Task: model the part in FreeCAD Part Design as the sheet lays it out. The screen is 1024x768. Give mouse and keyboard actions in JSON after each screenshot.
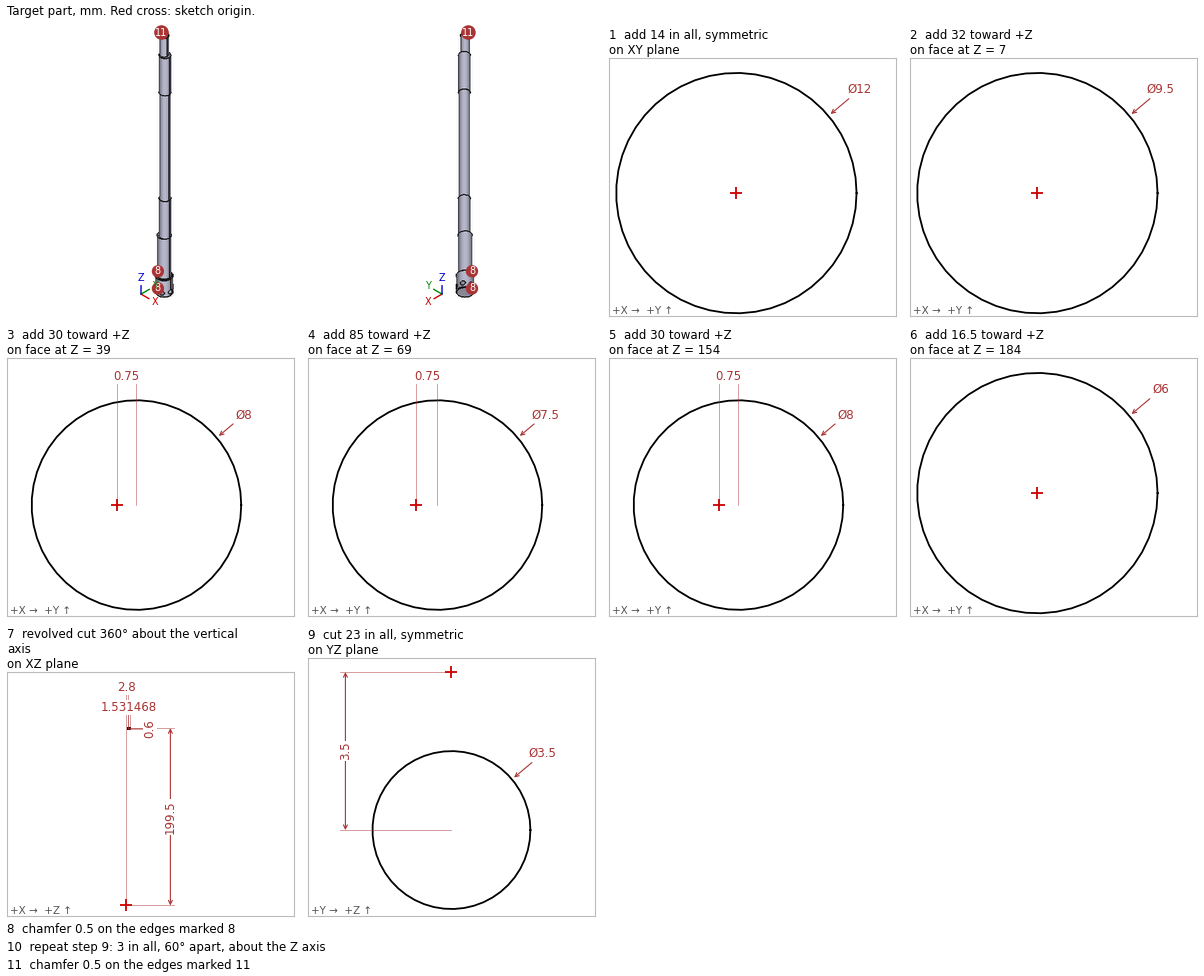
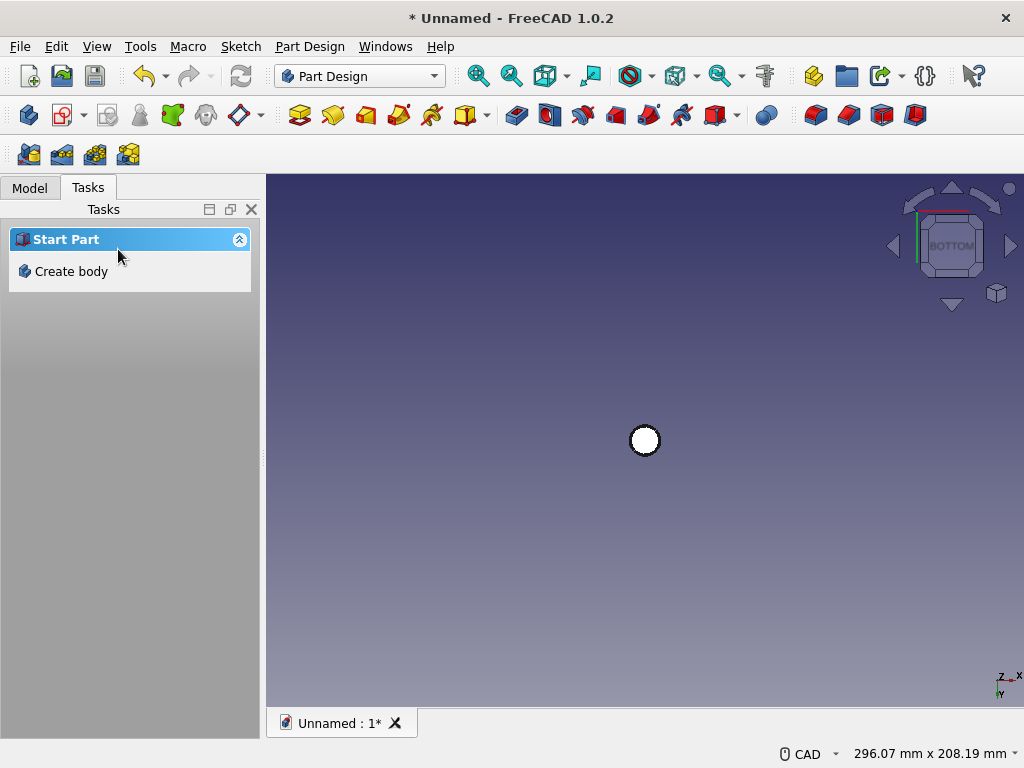
{"action": "key", "text": "v f"}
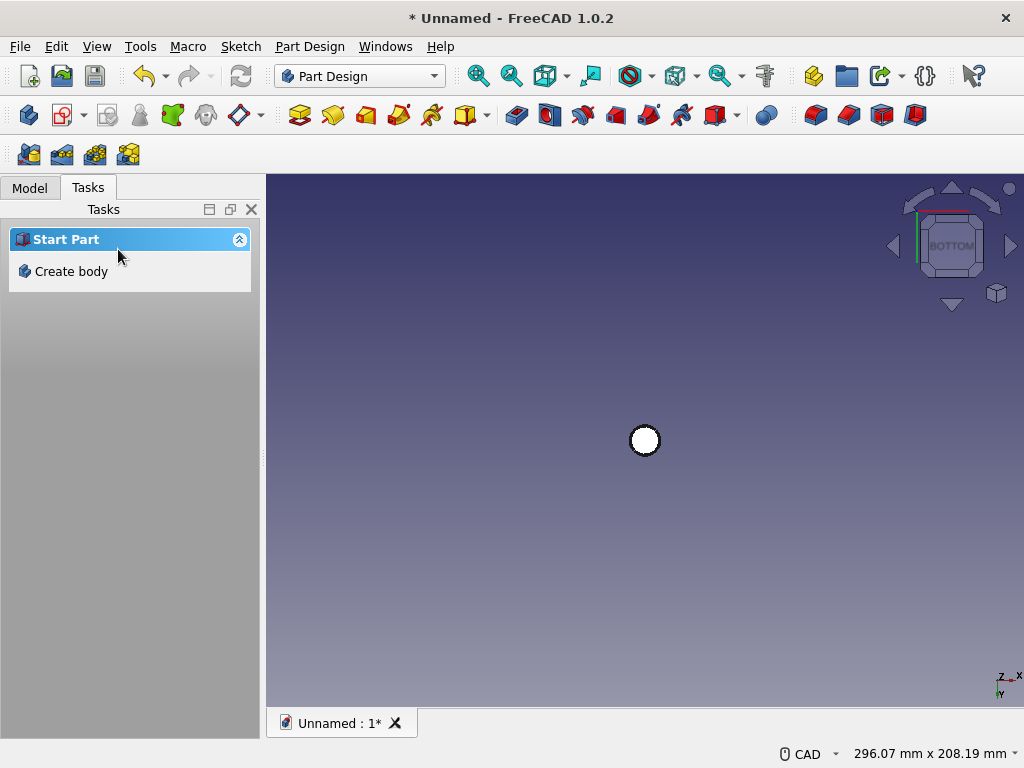
{"action": "left_click", "coordinate": [30, 188]}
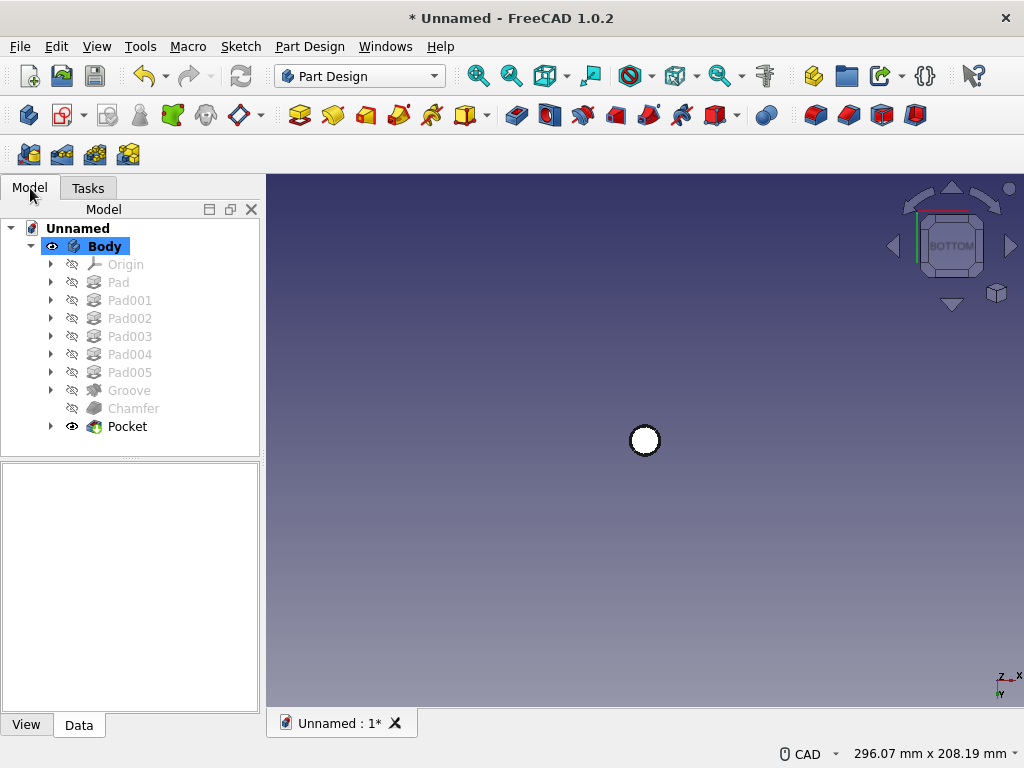
{"action": "left_click", "coordinate": [117, 426]}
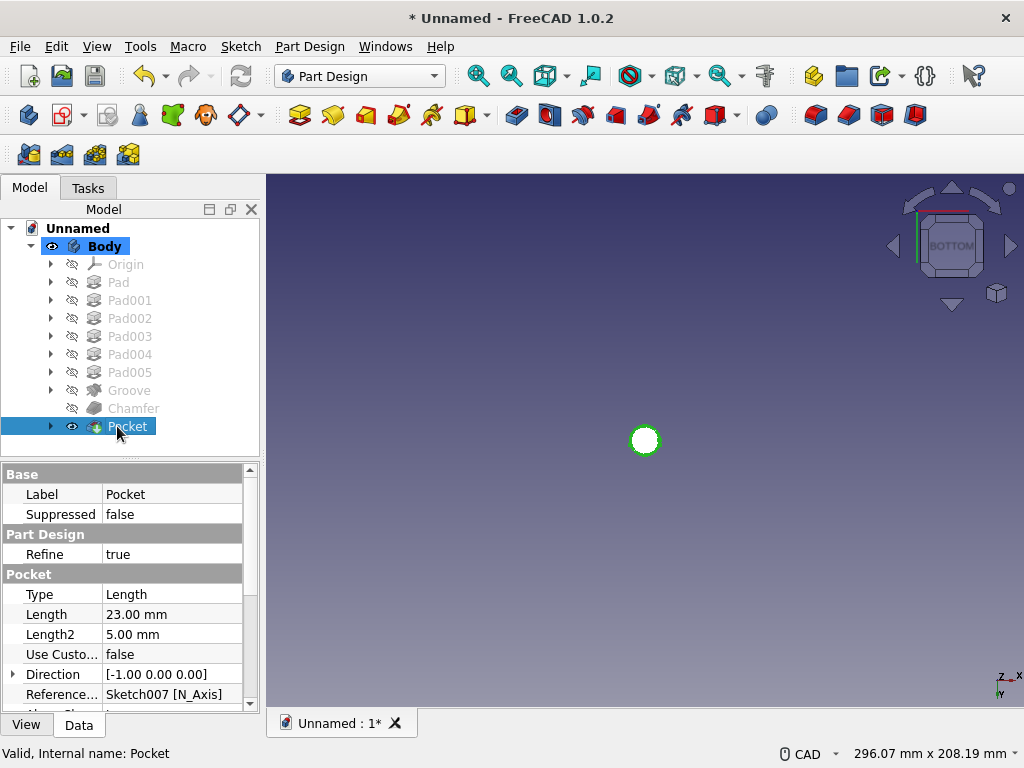
{"action": "left_click", "coordinate": [95, 154]}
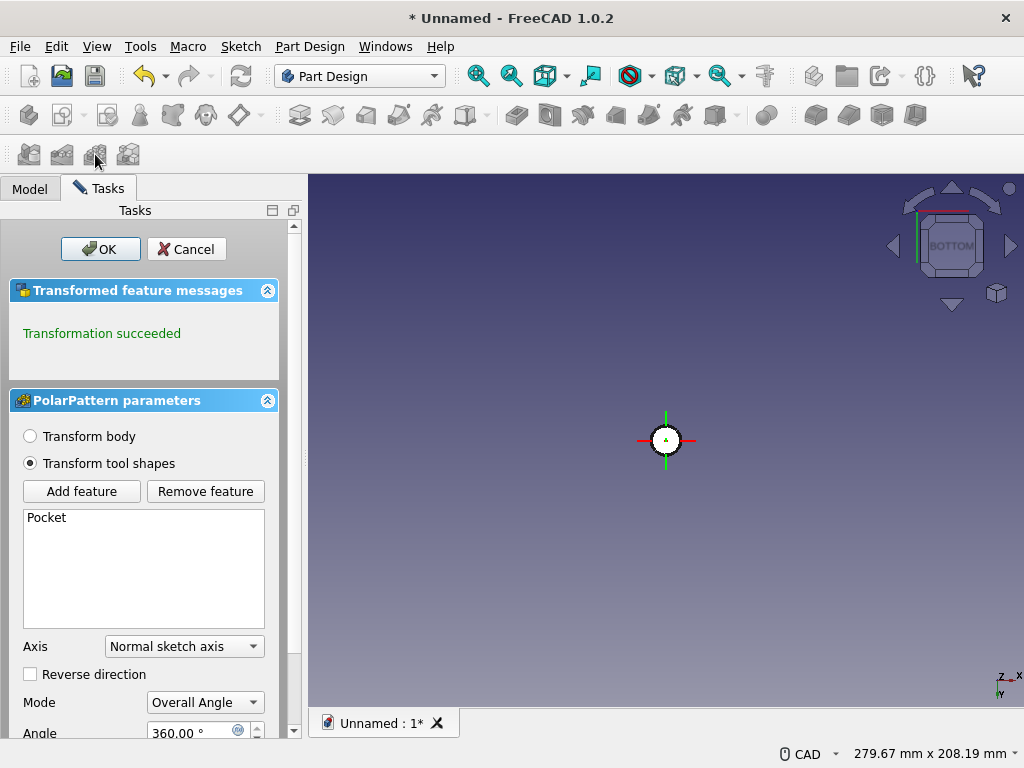
{"action": "left_click", "coordinate": [185, 646]}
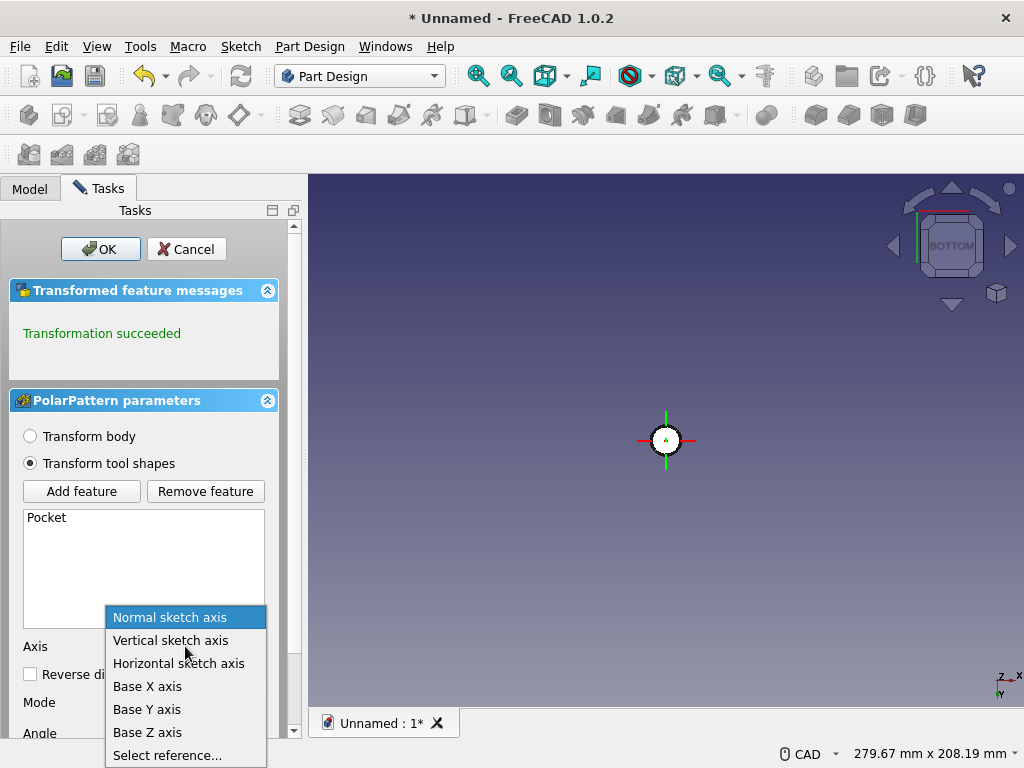
{"action": "left_click", "coordinate": [184, 732]}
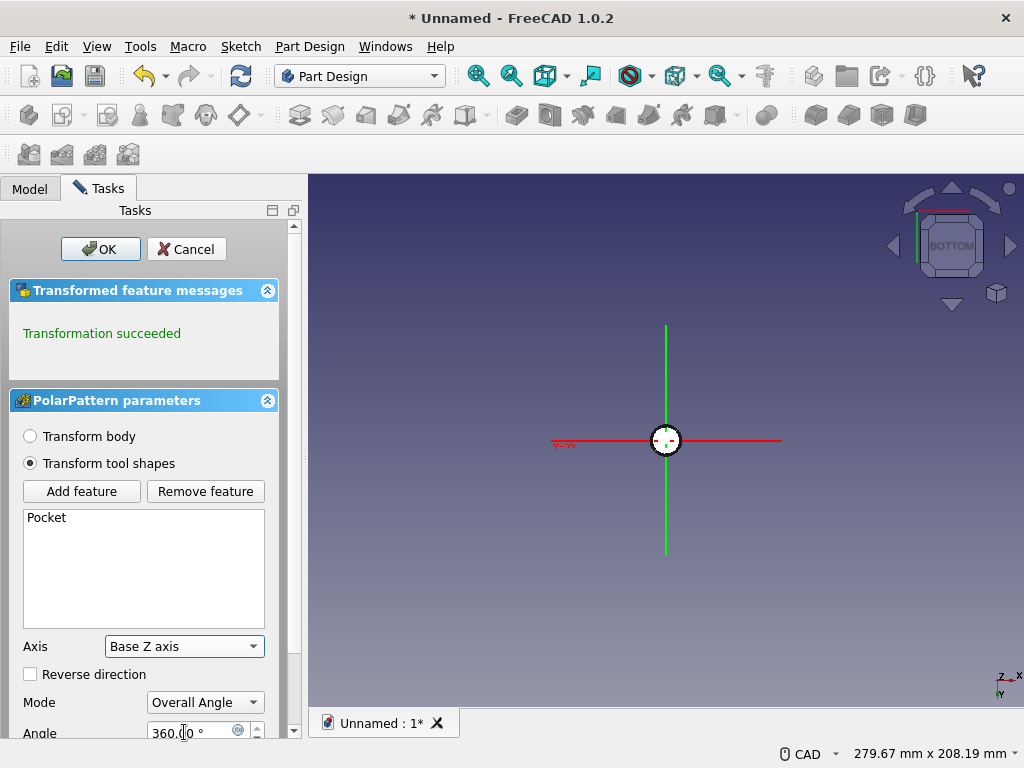
{"action": "left_click", "coordinate": [206, 702]}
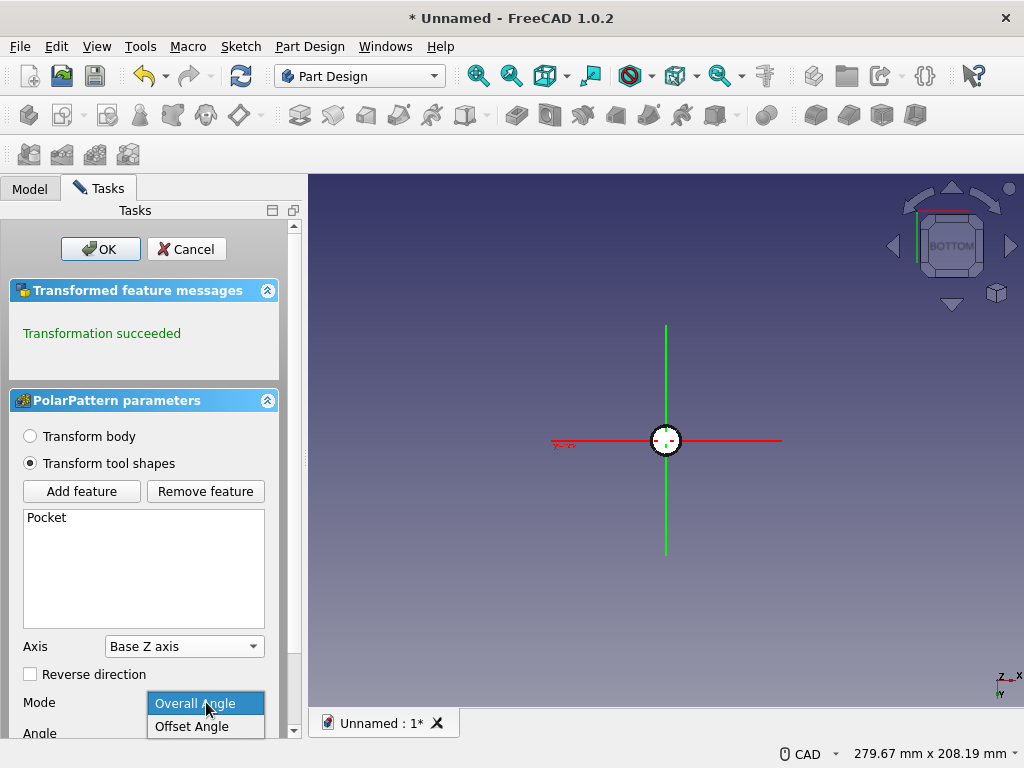
{"action": "left_click", "coordinate": [204, 726]}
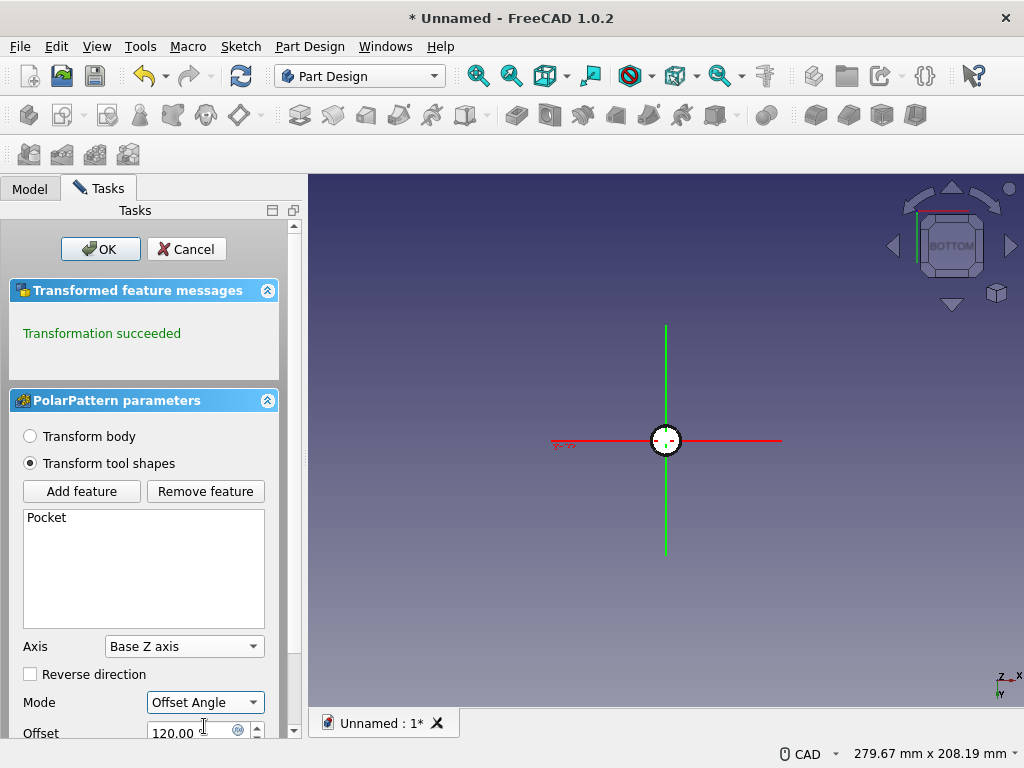
{"action": "scroll", "coordinate": [294, 479], "scroll_direction": "down", "scroll_amount": 2}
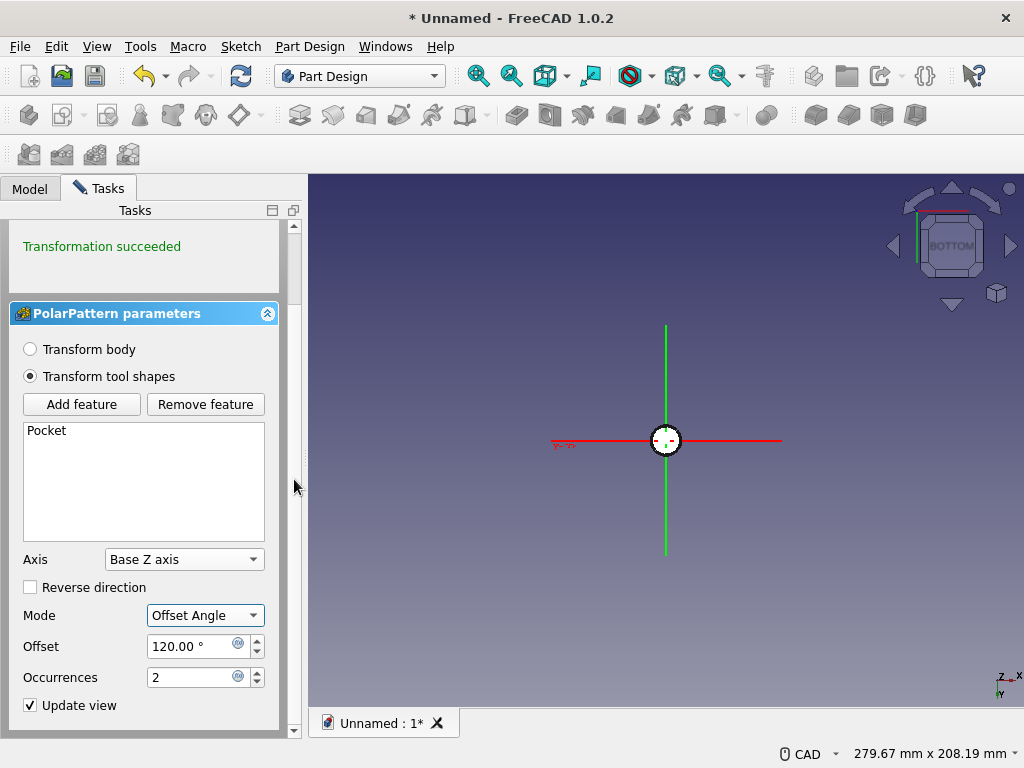
{"action": "triple_click", "coordinate": [199, 646]}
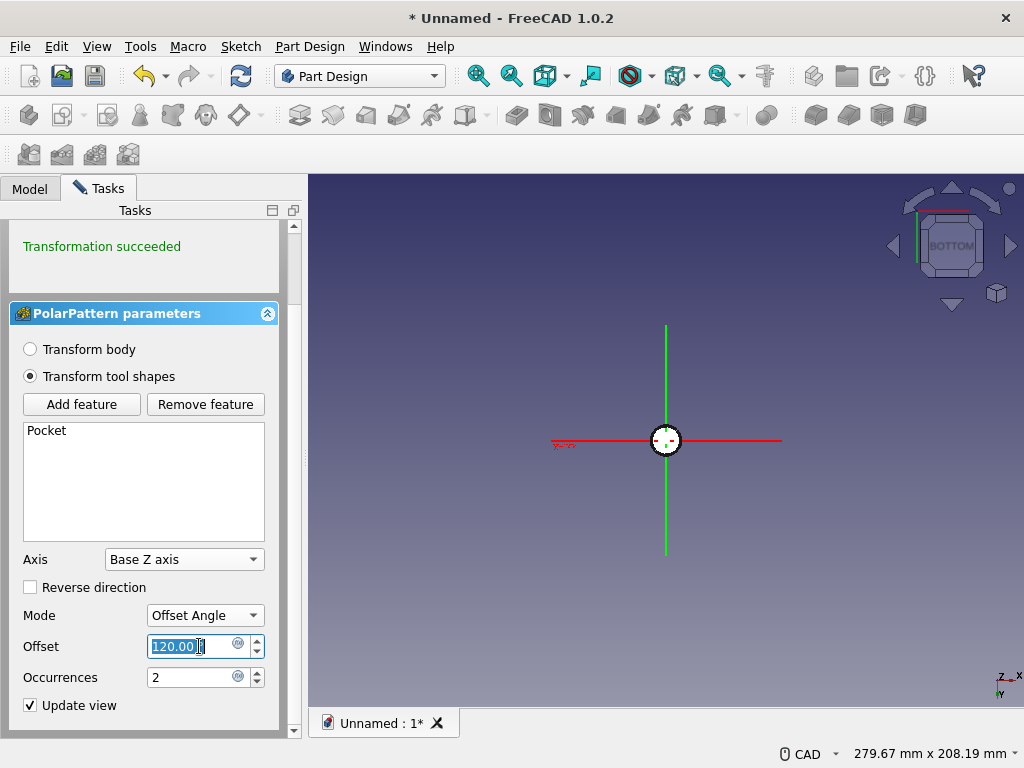
{"action": "type", "text": "60"}
{"action": "key", "text": "Tab"}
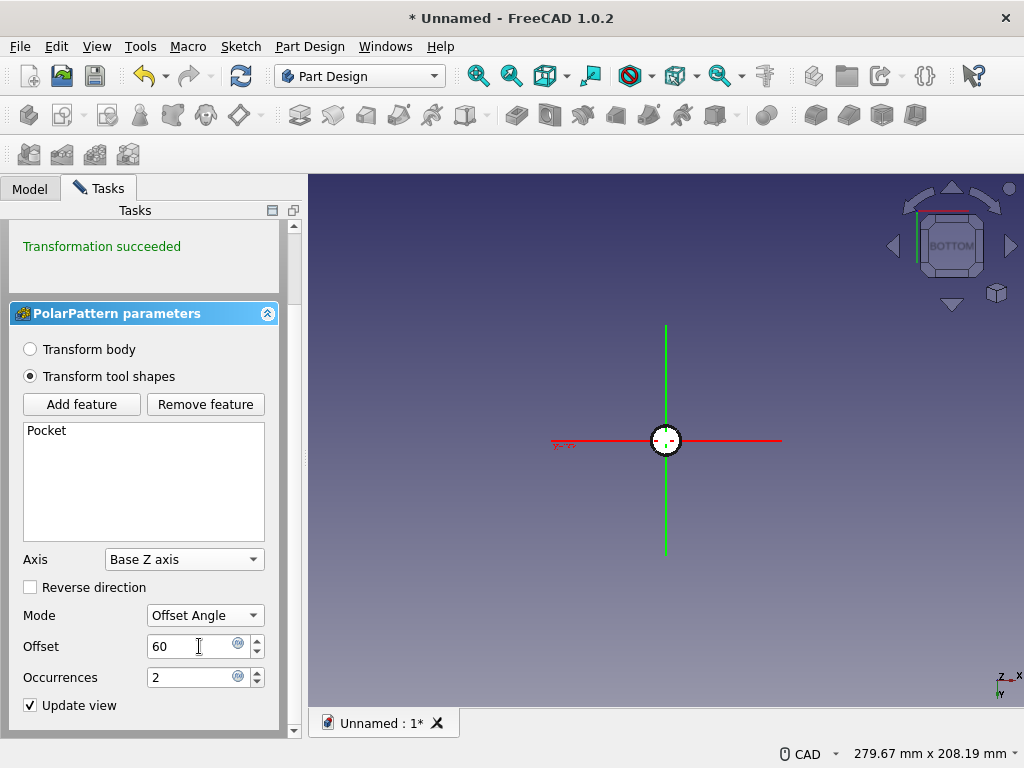
{"action": "triple_click", "coordinate": [199, 678]}